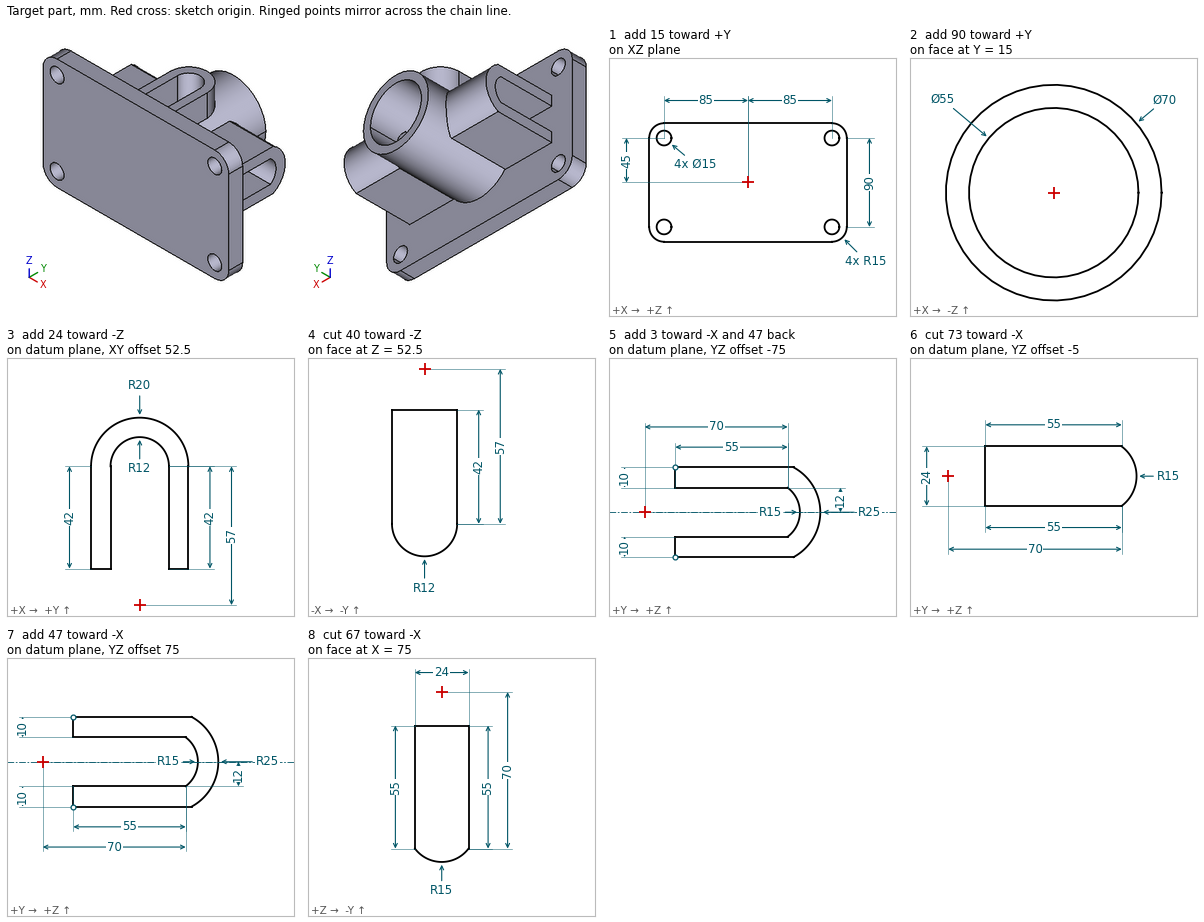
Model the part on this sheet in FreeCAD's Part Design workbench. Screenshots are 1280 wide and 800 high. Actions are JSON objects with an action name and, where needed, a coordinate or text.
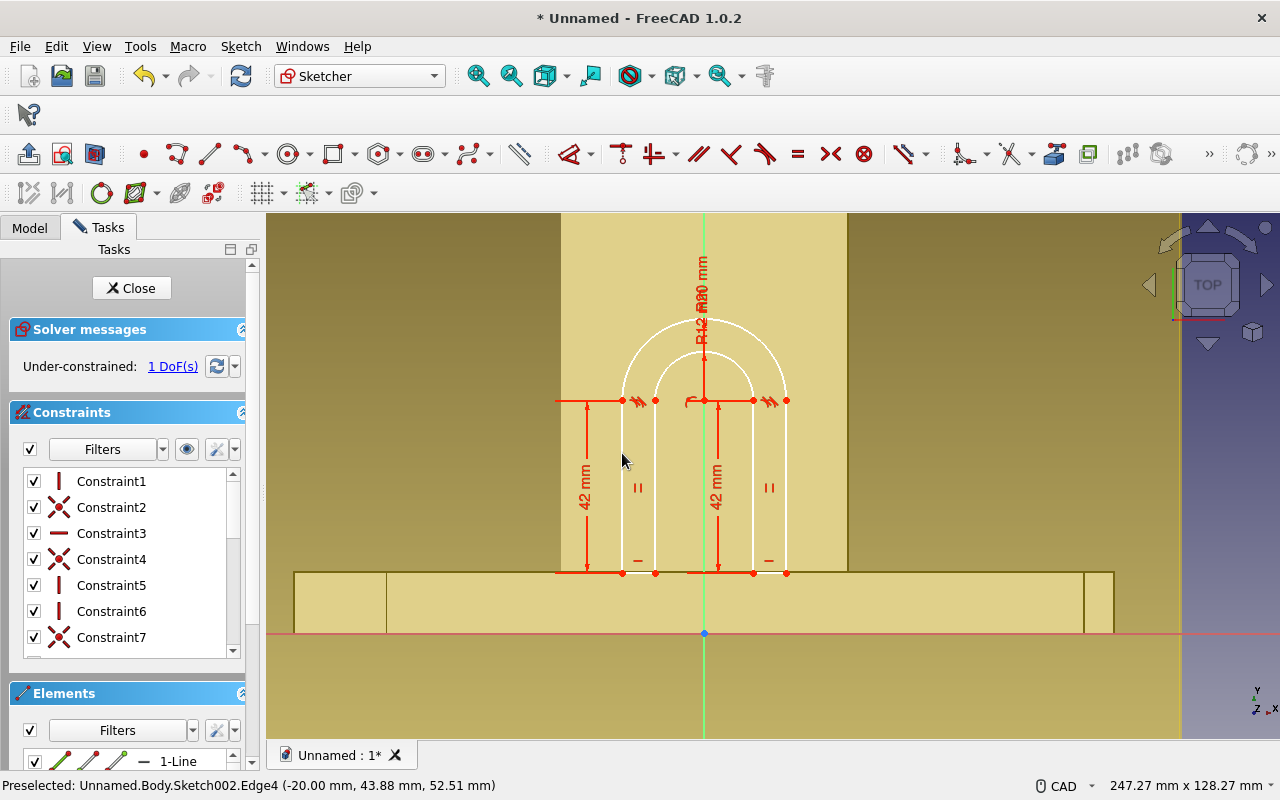
{"action": "left_click", "coordinate": [753, 401]}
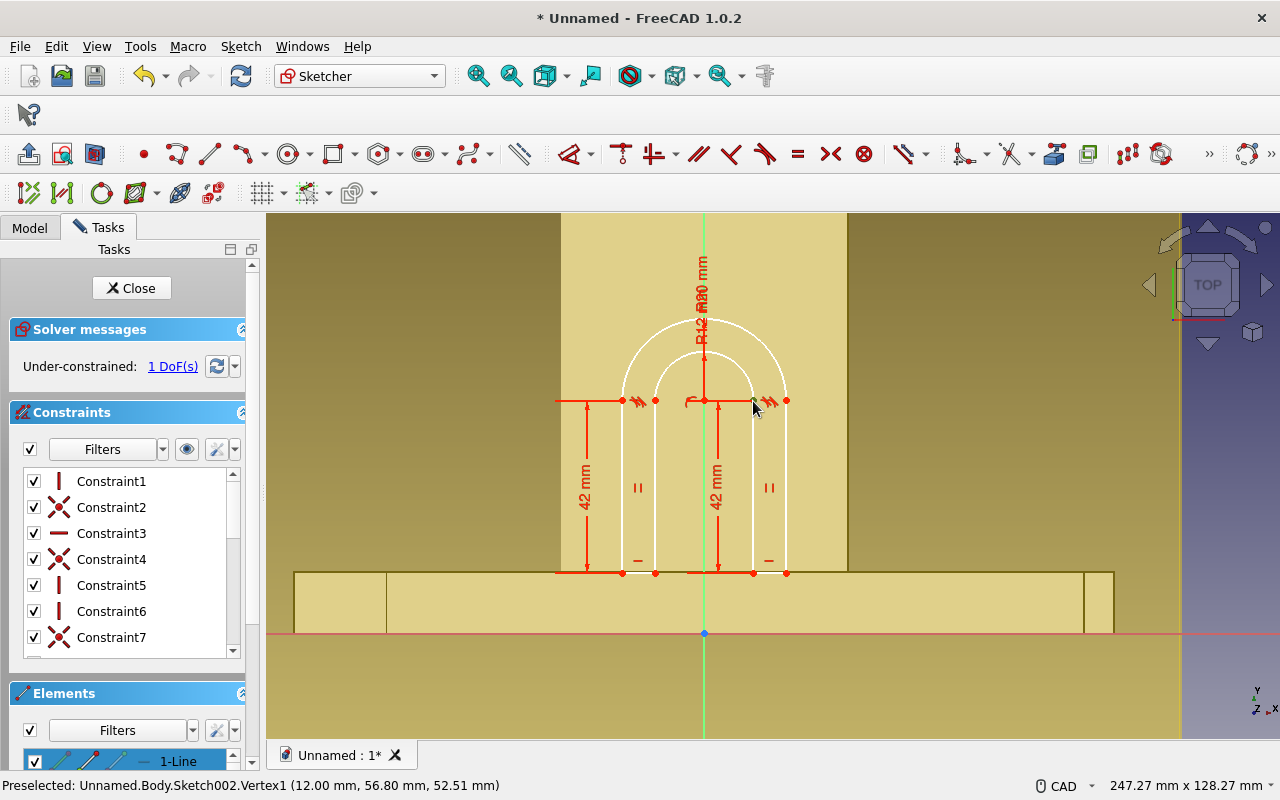
{"action": "key", "text": "i"}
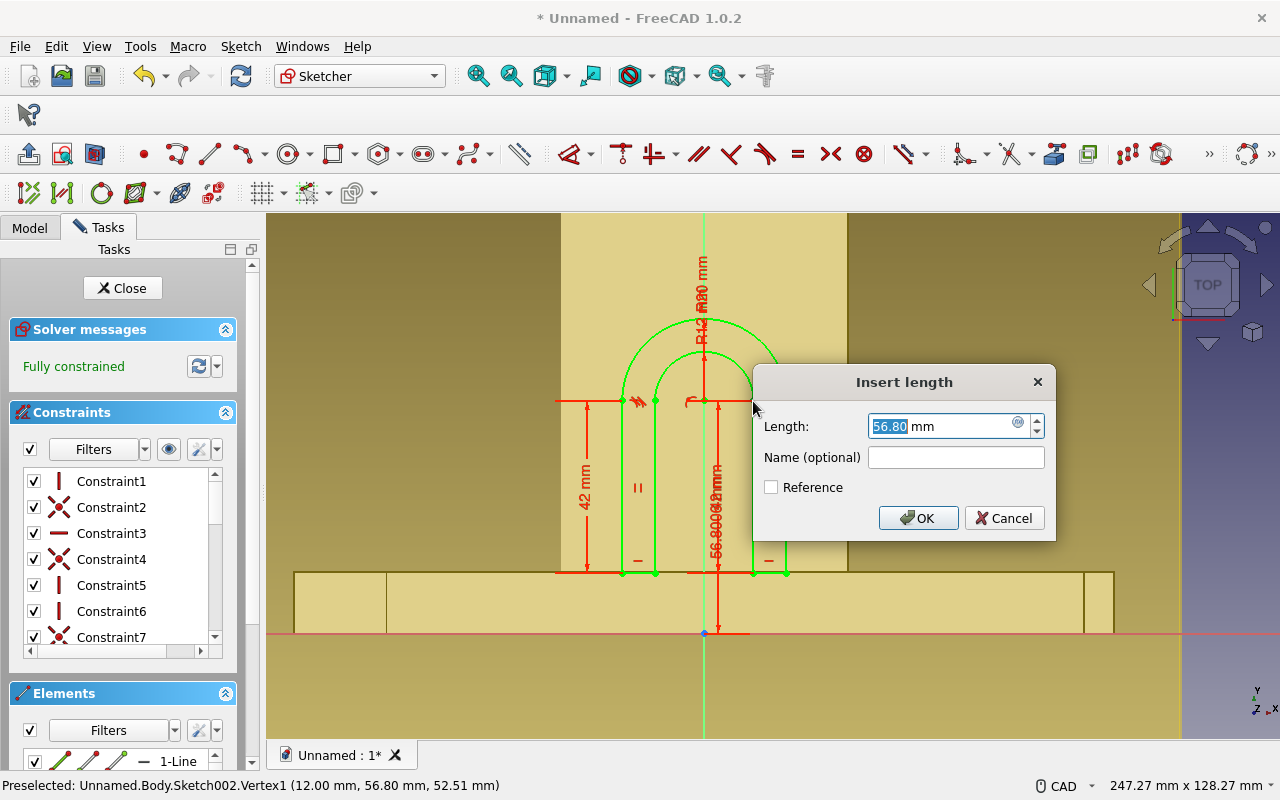
{"action": "type", "text": "57"}
{"action": "key", "text": "Return"}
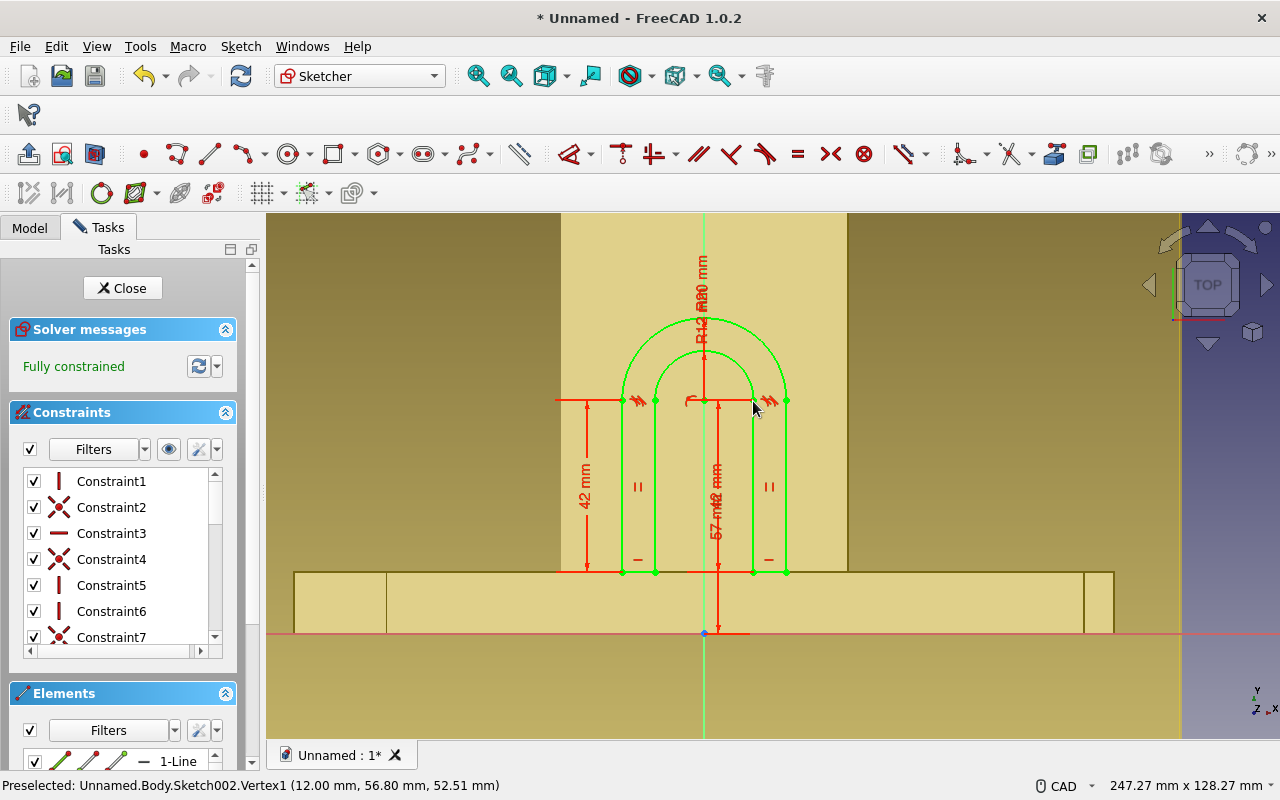
{"action": "left_click", "coordinate": [123, 288]}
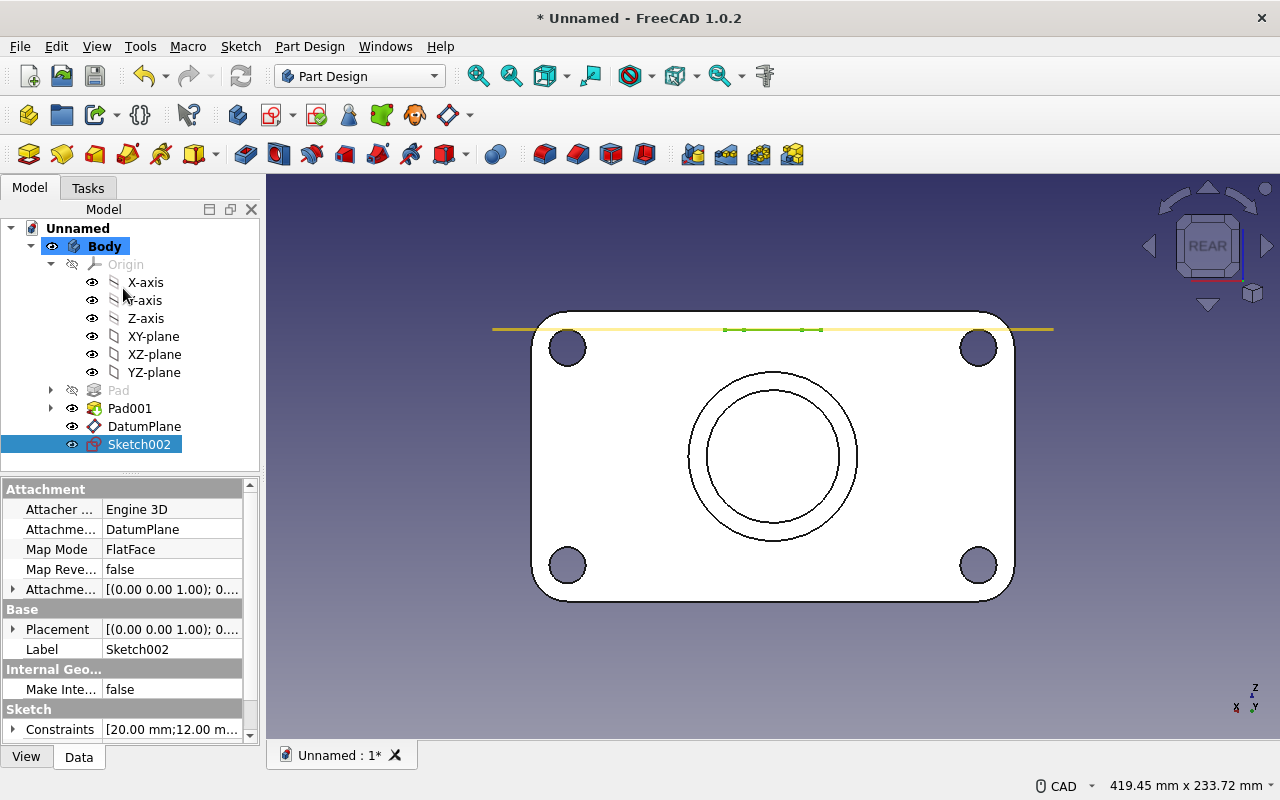
{"action": "left_click", "coordinate": [29, 154]}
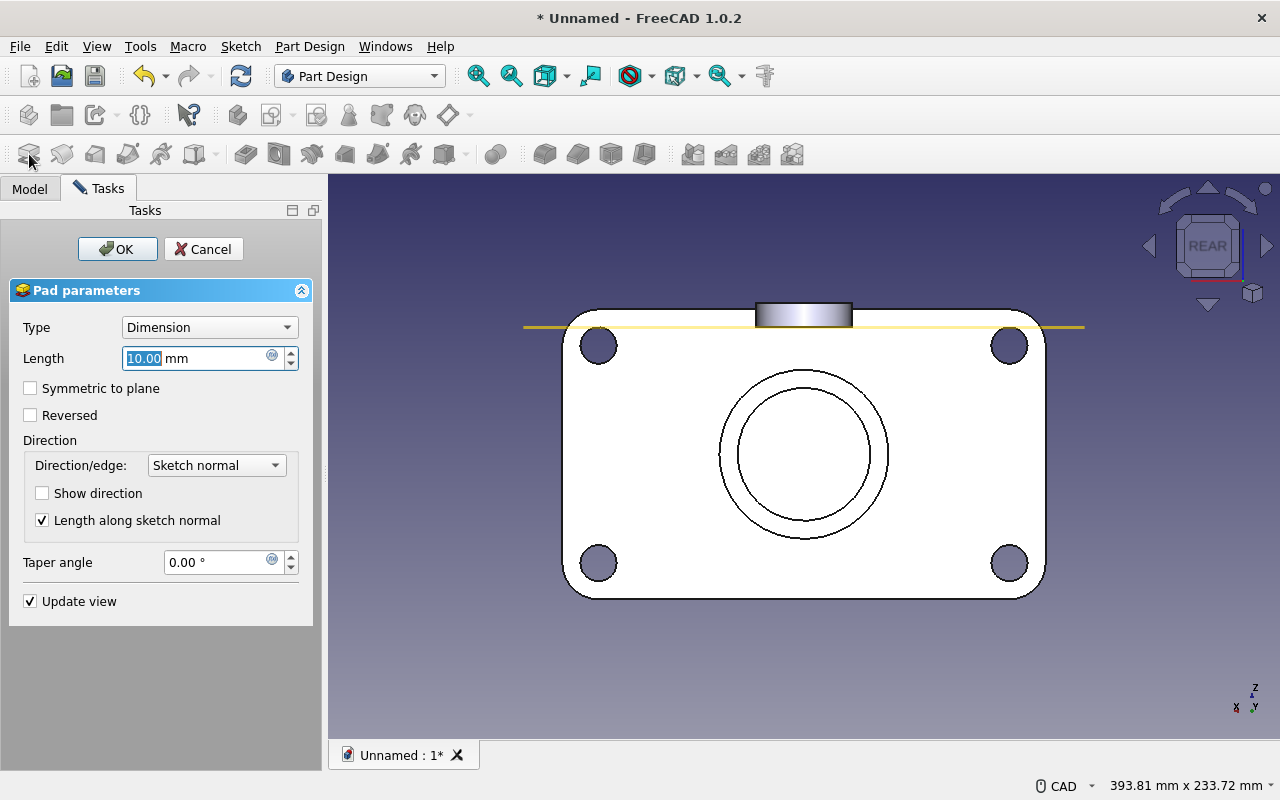
{"action": "type", "text": "24"}
{"action": "key", "text": "Tab"}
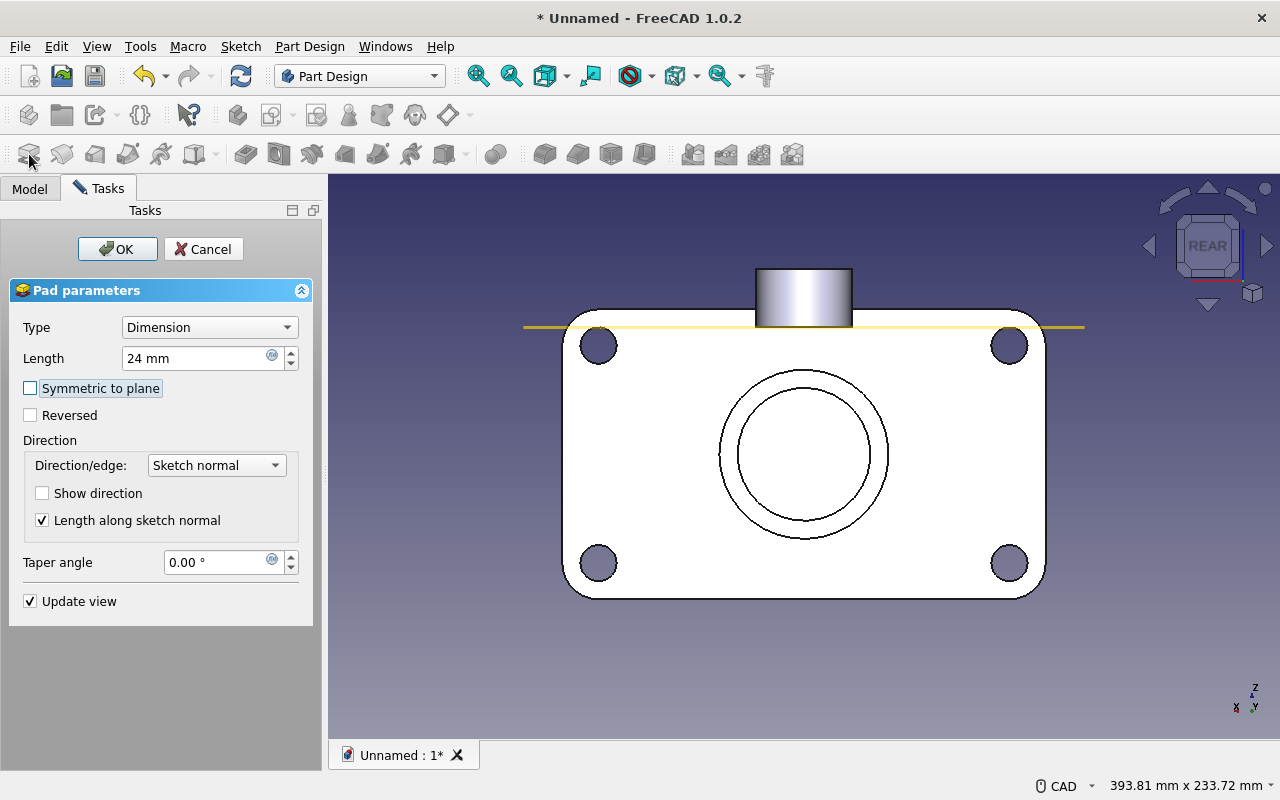
{"action": "left_click", "coordinate": [31, 415]}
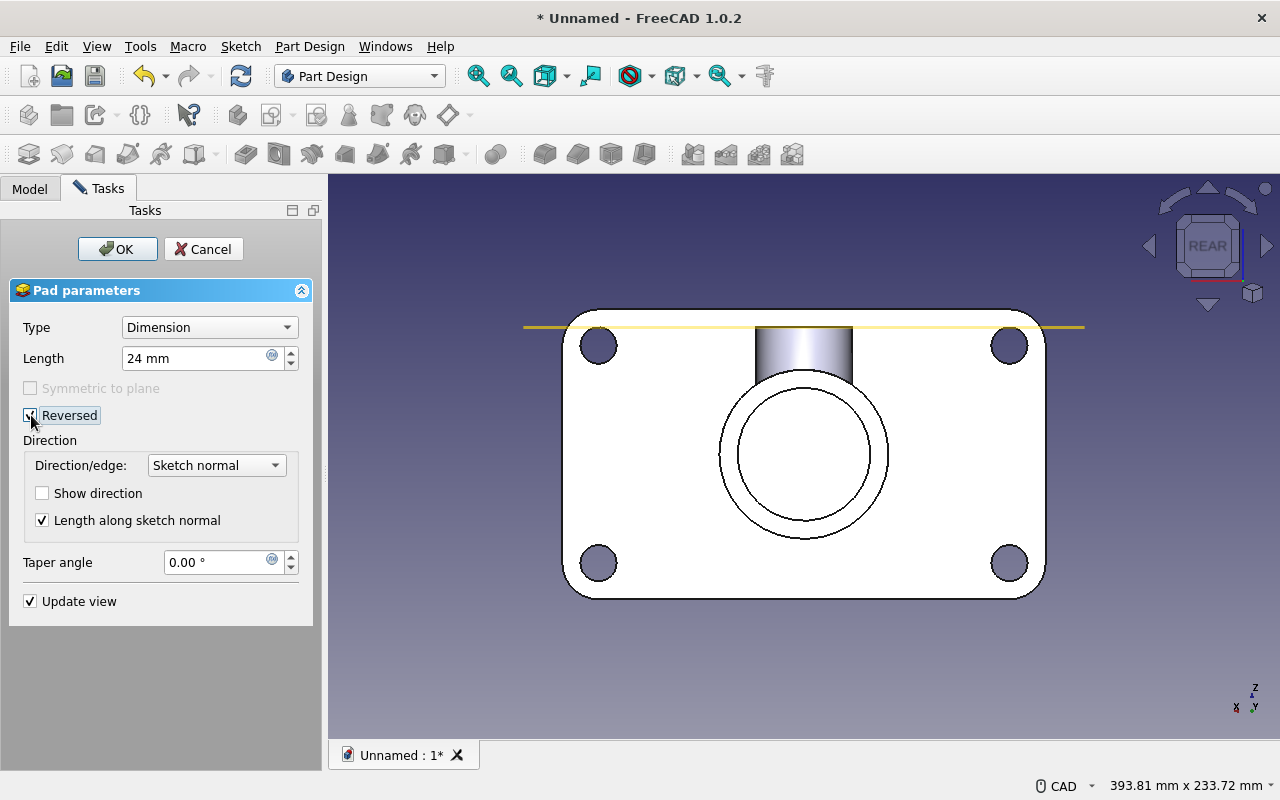
{"action": "left_click", "coordinate": [118, 249]}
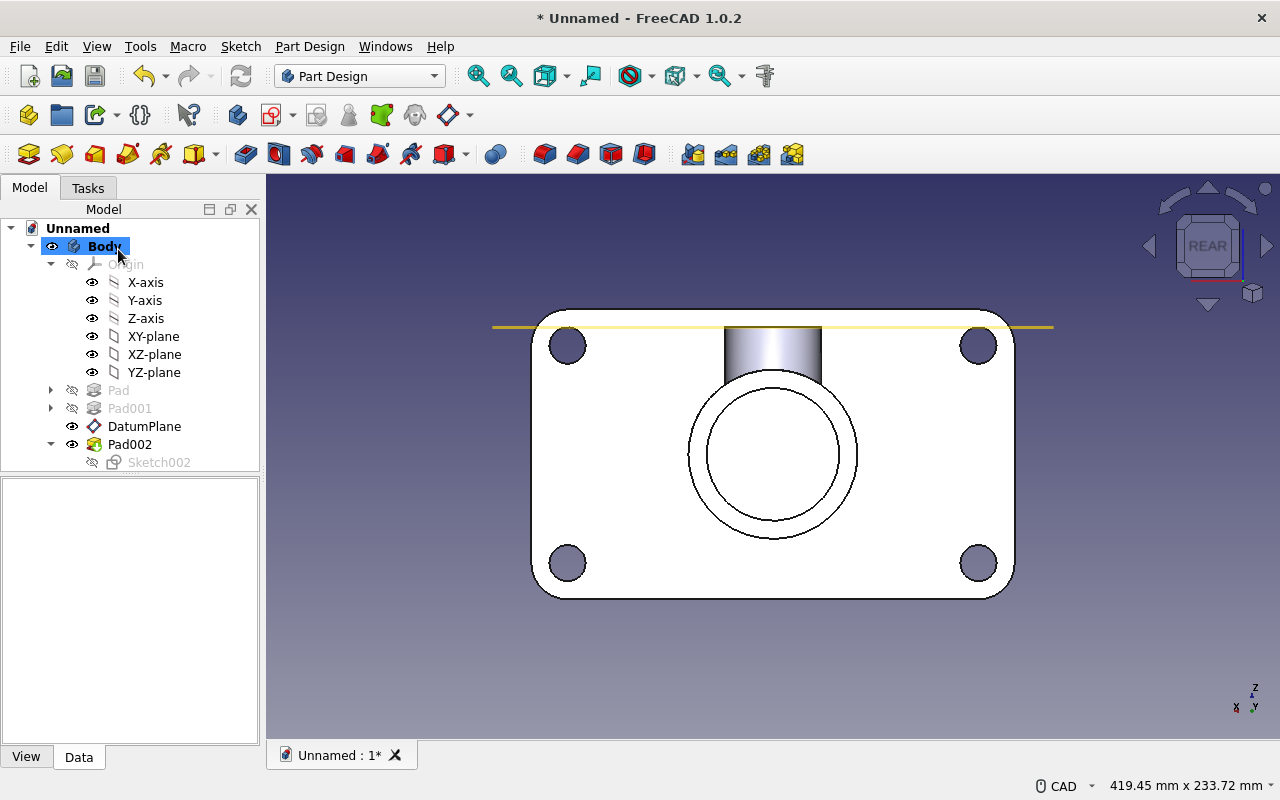
{"action": "left_click", "coordinate": [117, 426]}
{"action": "key", "text": "space"}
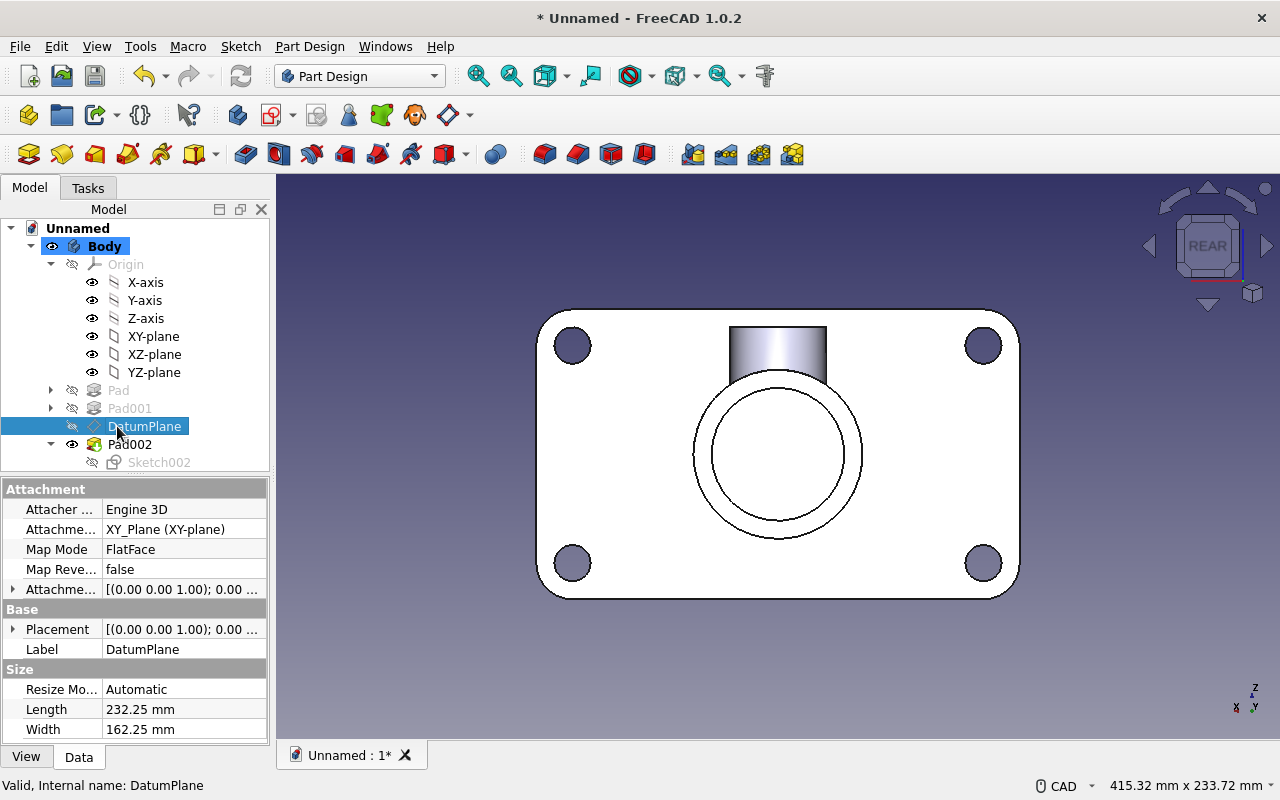
{"action": "key", "text": "0"}